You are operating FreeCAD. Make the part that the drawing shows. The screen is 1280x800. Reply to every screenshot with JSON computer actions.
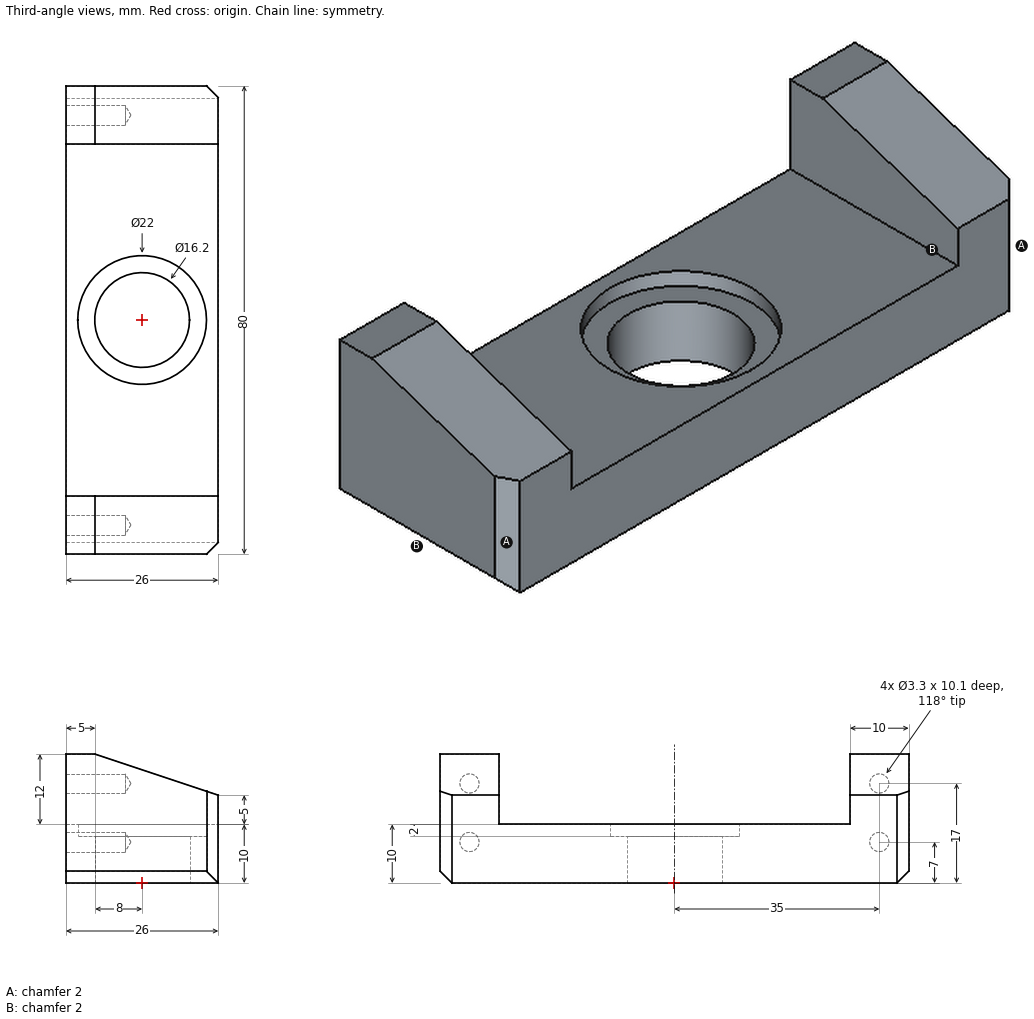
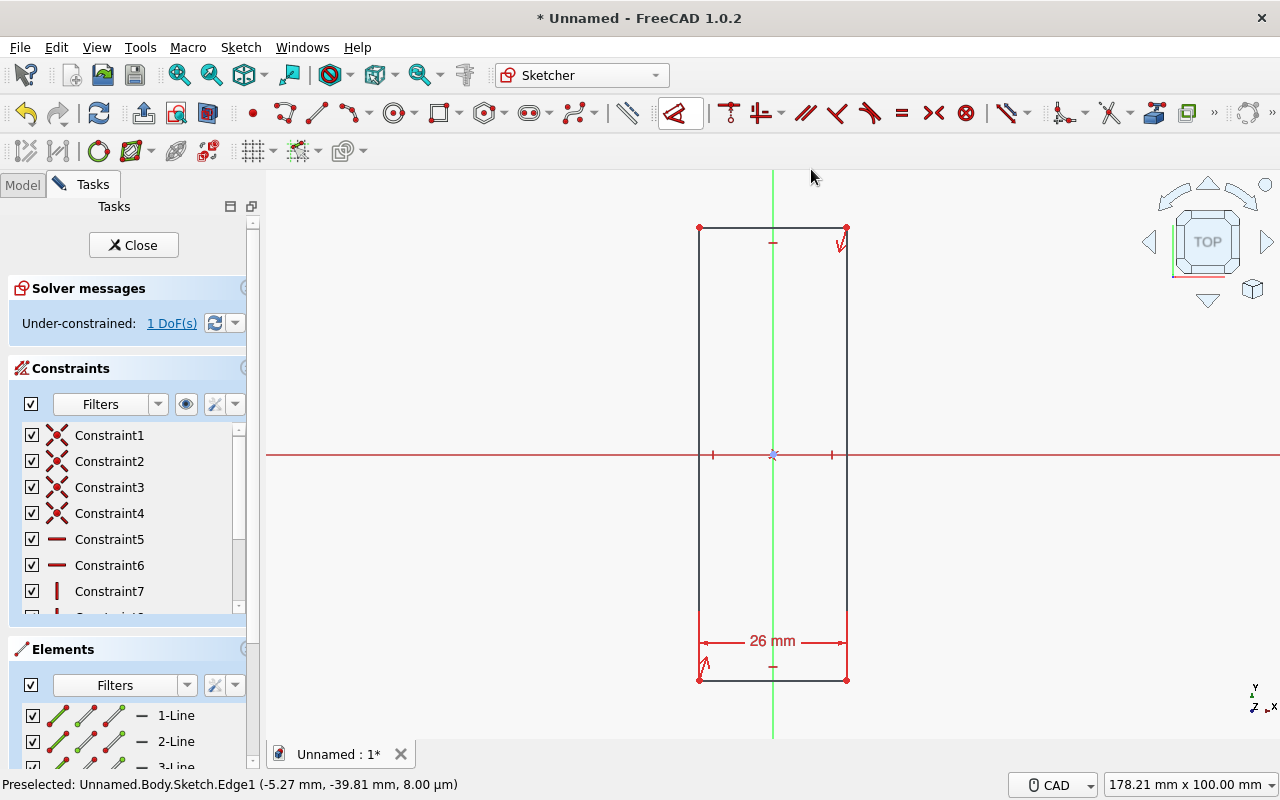
{"action": "left_click", "coordinate": [847, 545]}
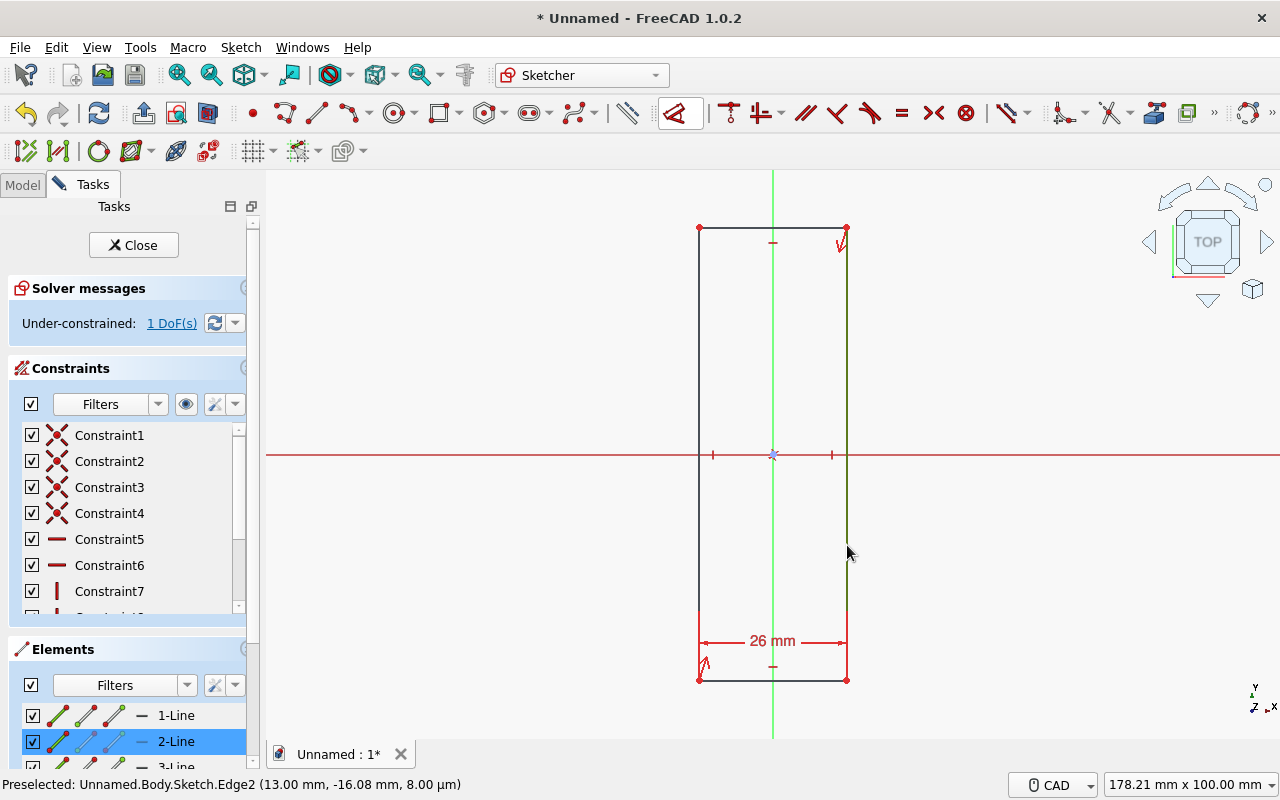
{"action": "left_click", "coordinate": [698, 114]}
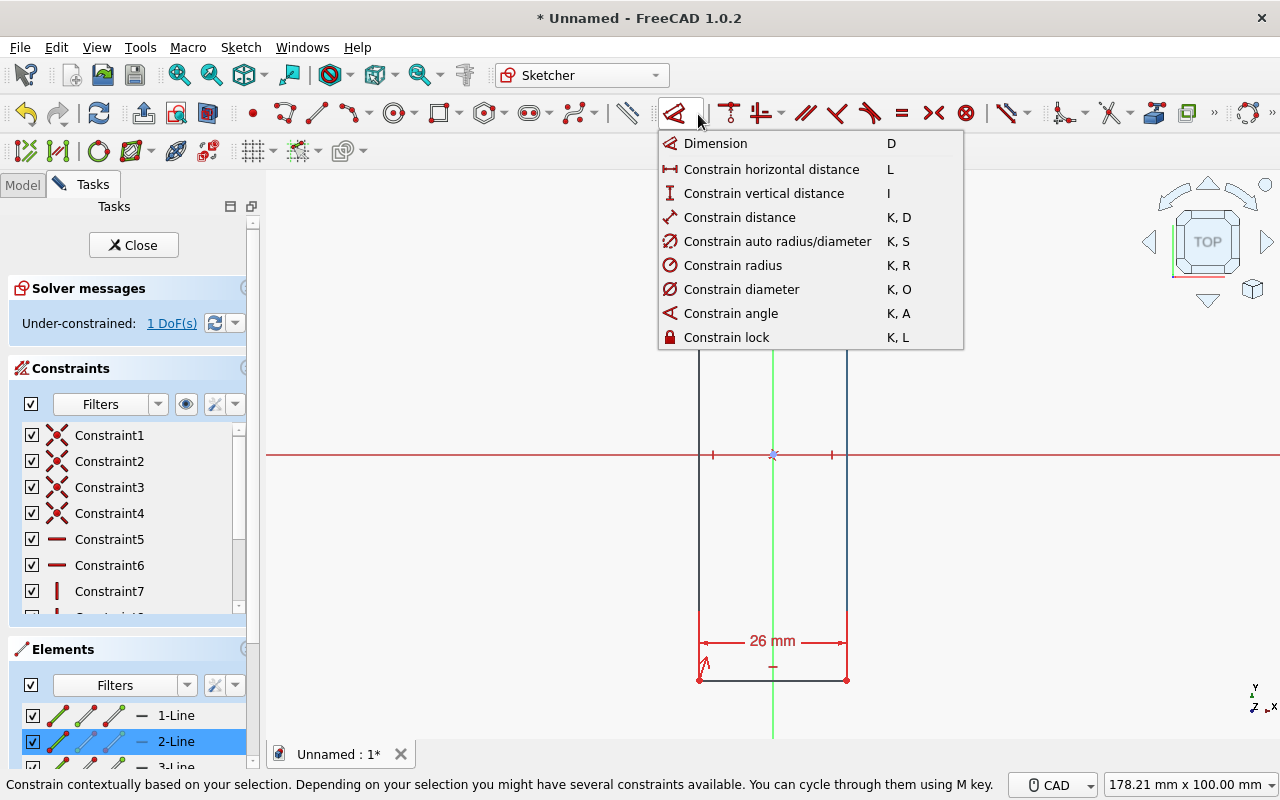
{"action": "left_click", "coordinate": [811, 193]}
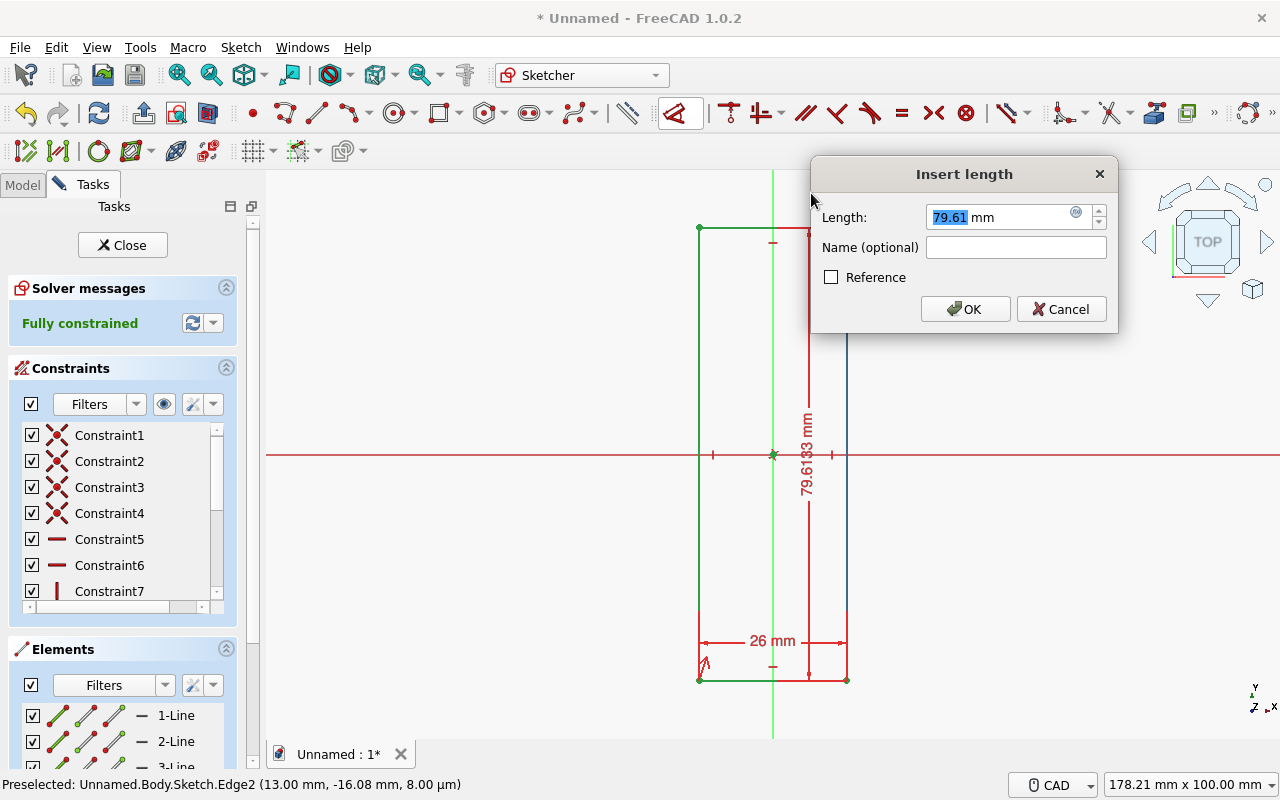
{"action": "type", "text": "80"}
{"action": "key", "text": "Return"}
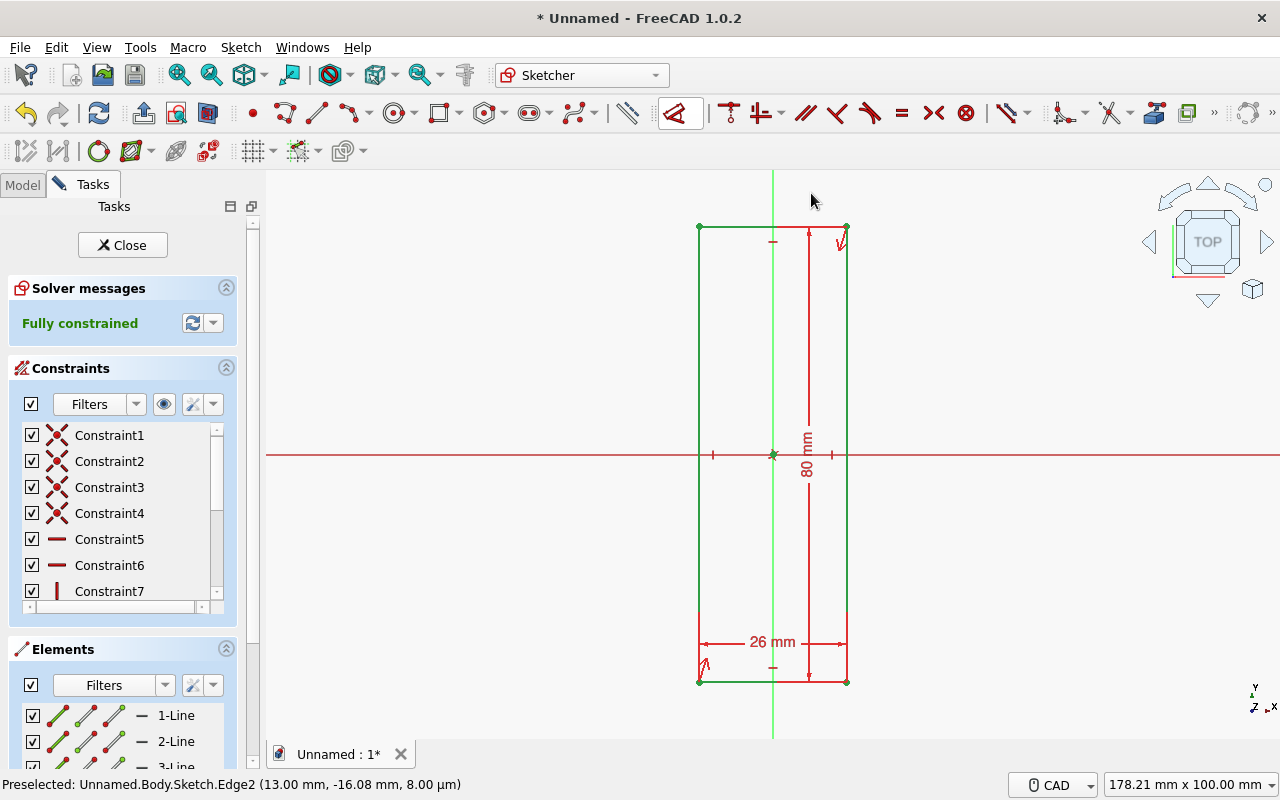
{"action": "left_click", "coordinate": [123, 245]}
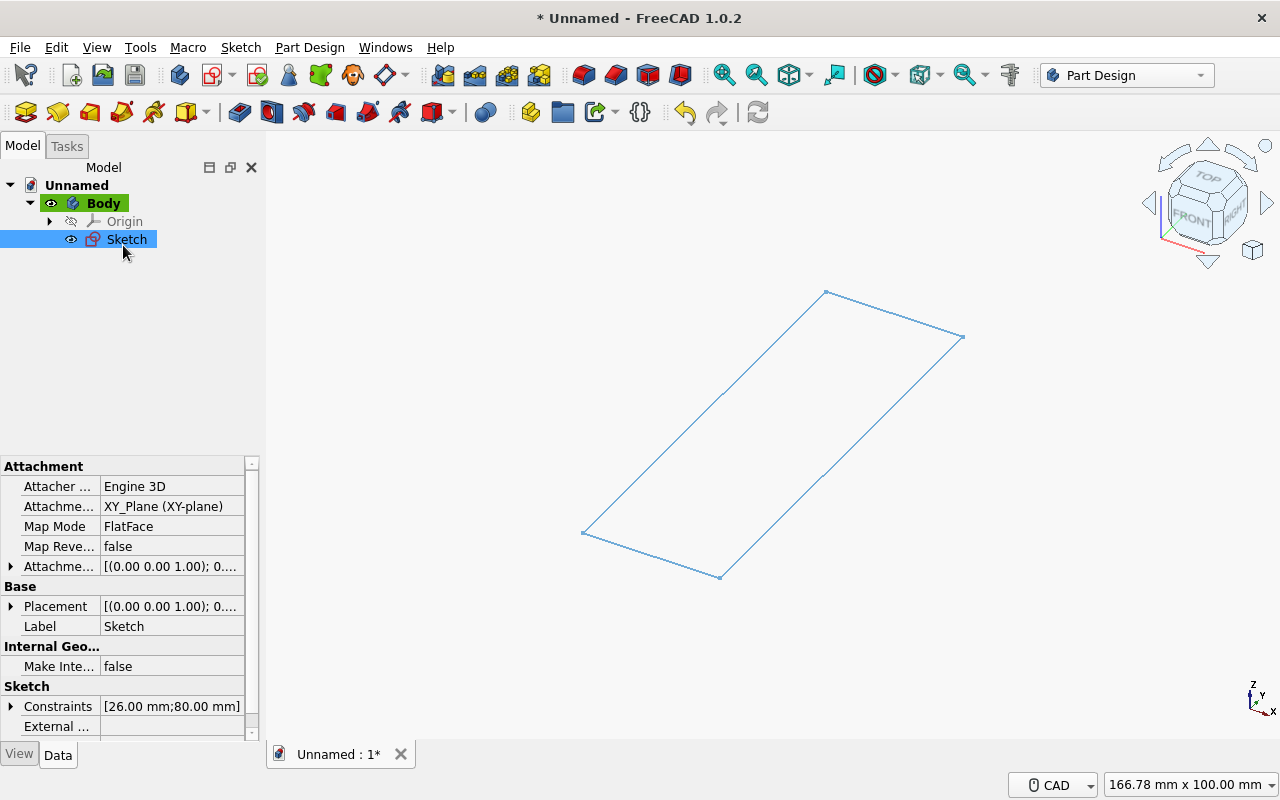
{"action": "left_click", "coordinate": [26, 112]}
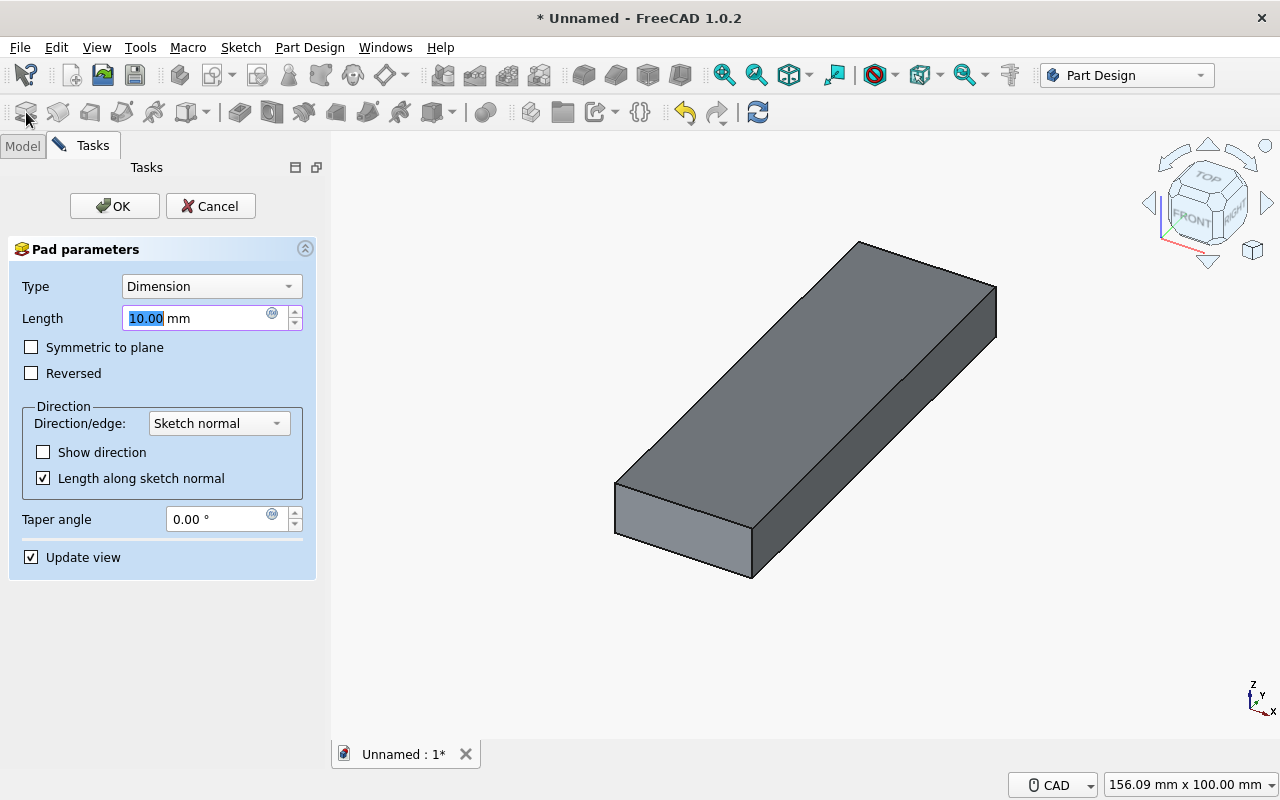
{"action": "type", "text": "10"}
{"action": "key", "text": "Tab"}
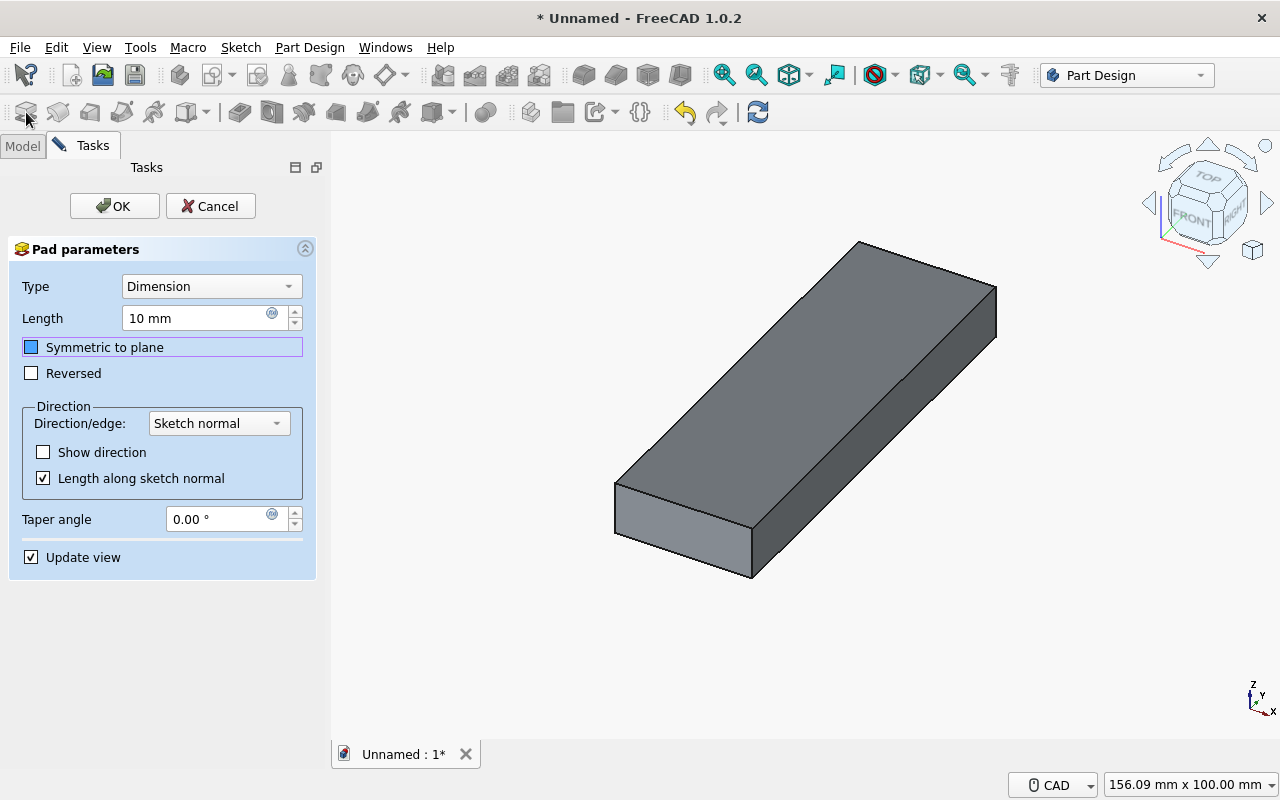
{"action": "left_click", "coordinate": [115, 206]}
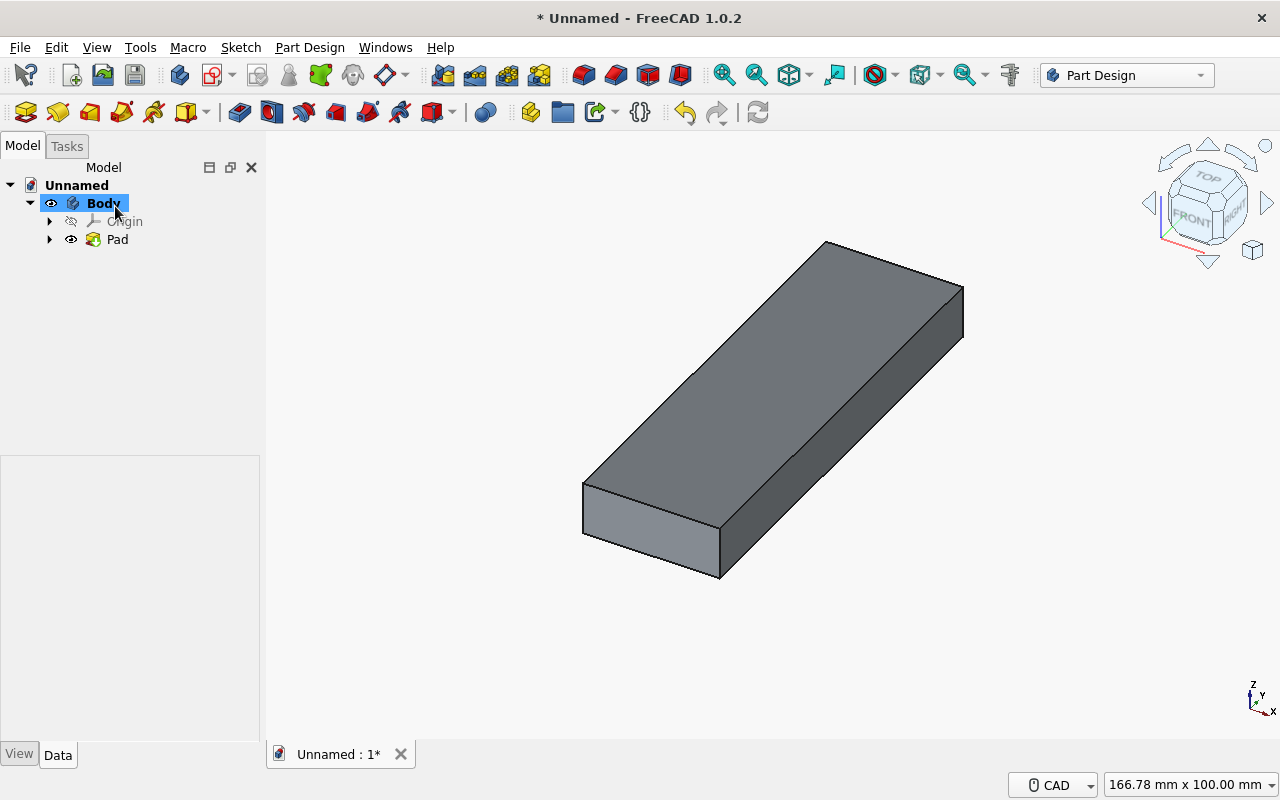
{"action": "left_click", "coordinate": [842, 315]}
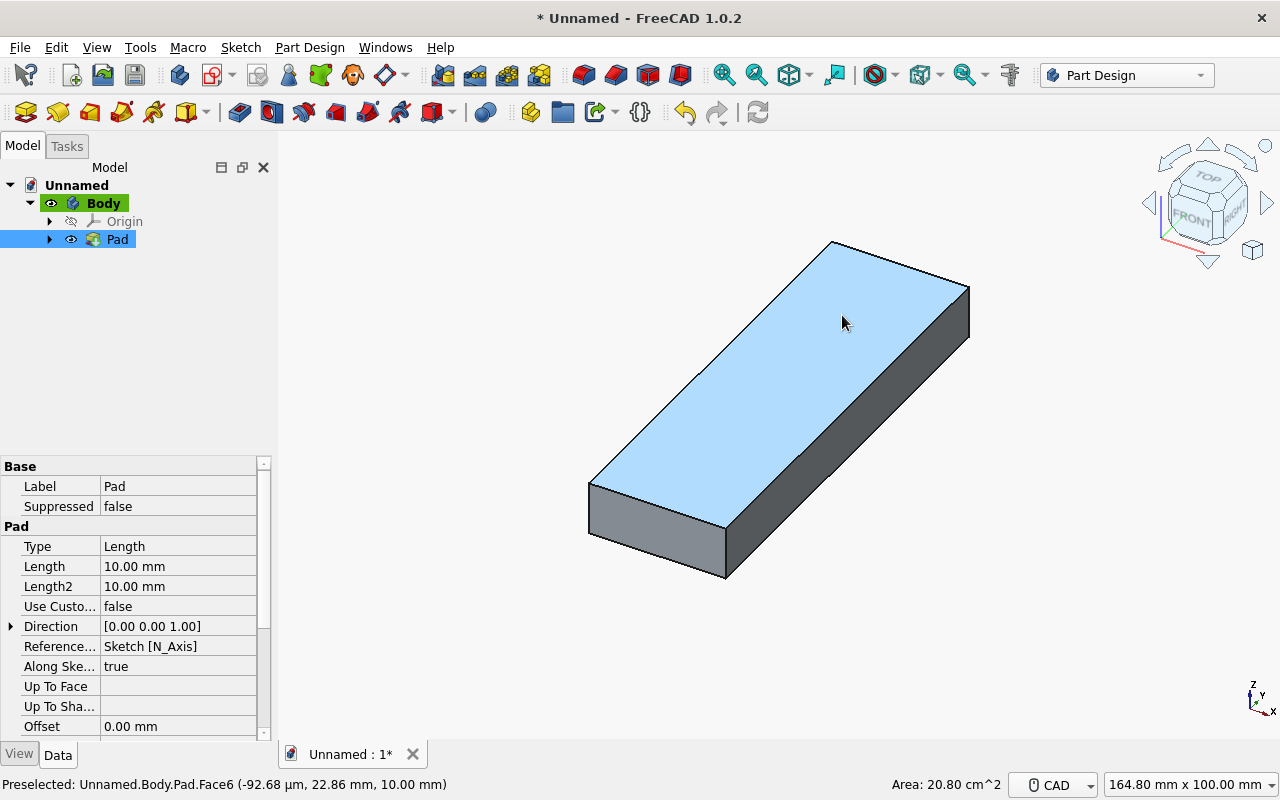
{"action": "left_click", "coordinate": [212, 76]}